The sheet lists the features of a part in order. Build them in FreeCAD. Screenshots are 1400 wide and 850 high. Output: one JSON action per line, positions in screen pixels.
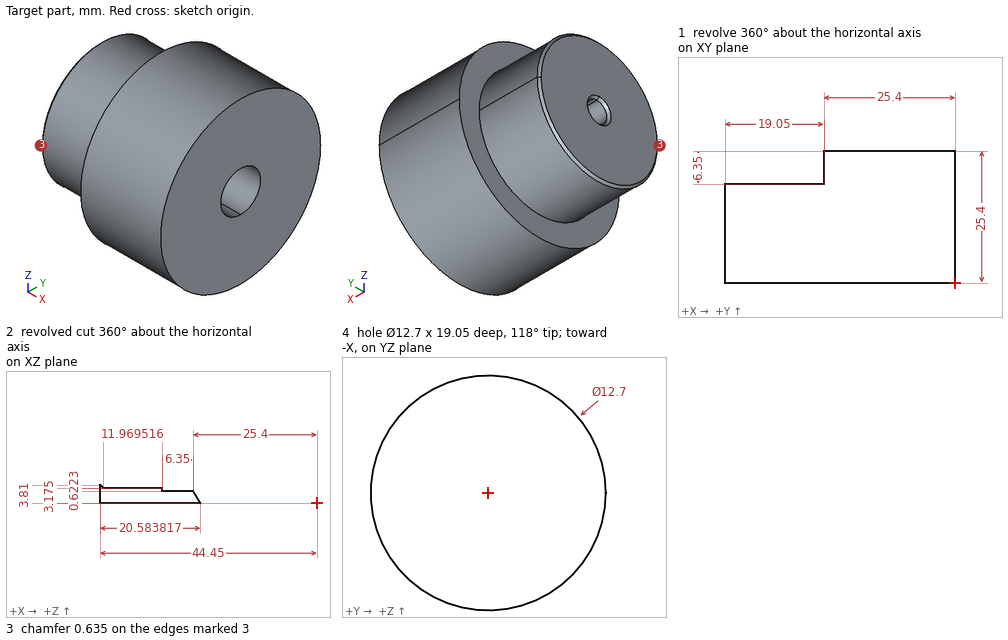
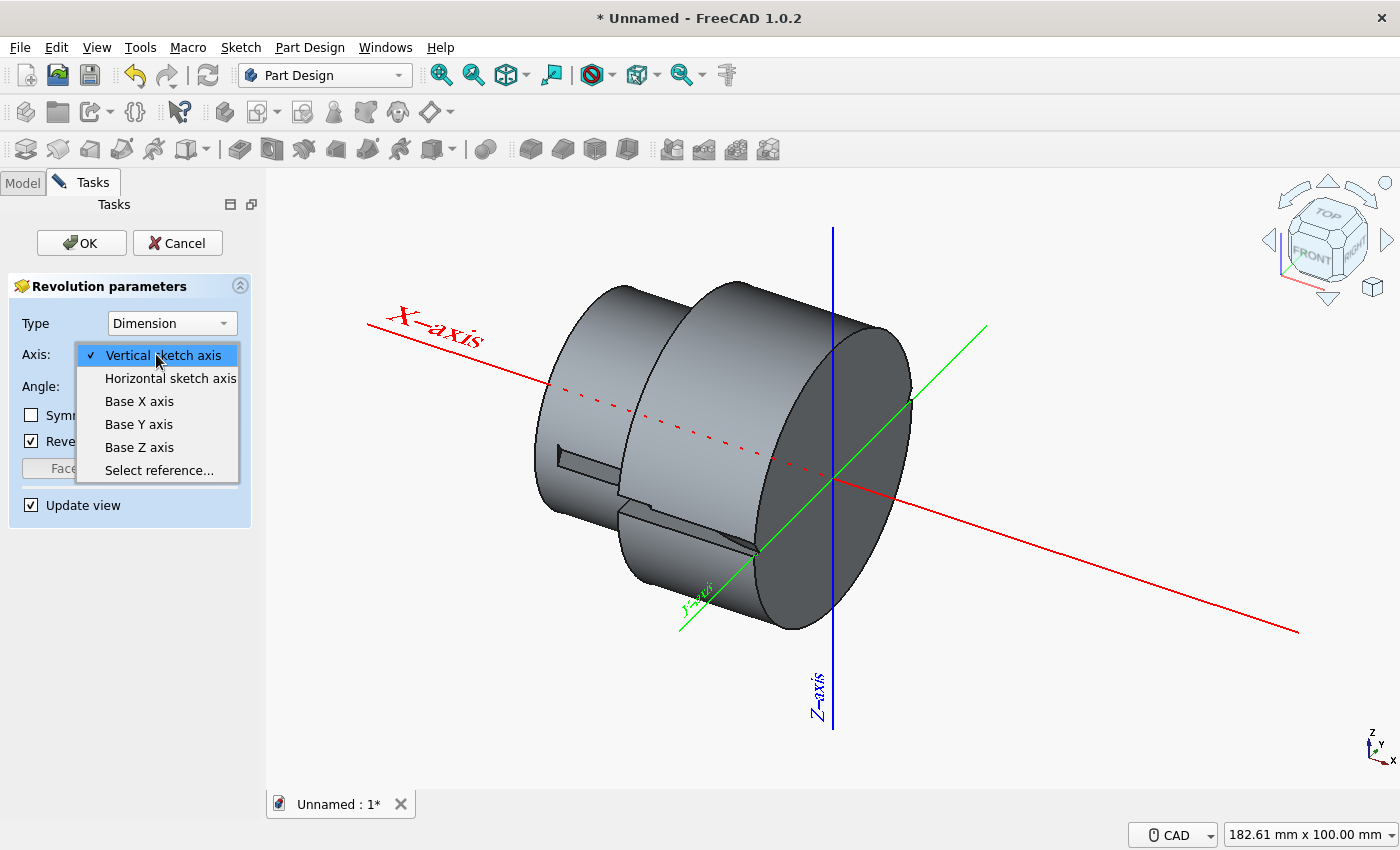
{"action": "left_click", "coordinate": [156, 378]}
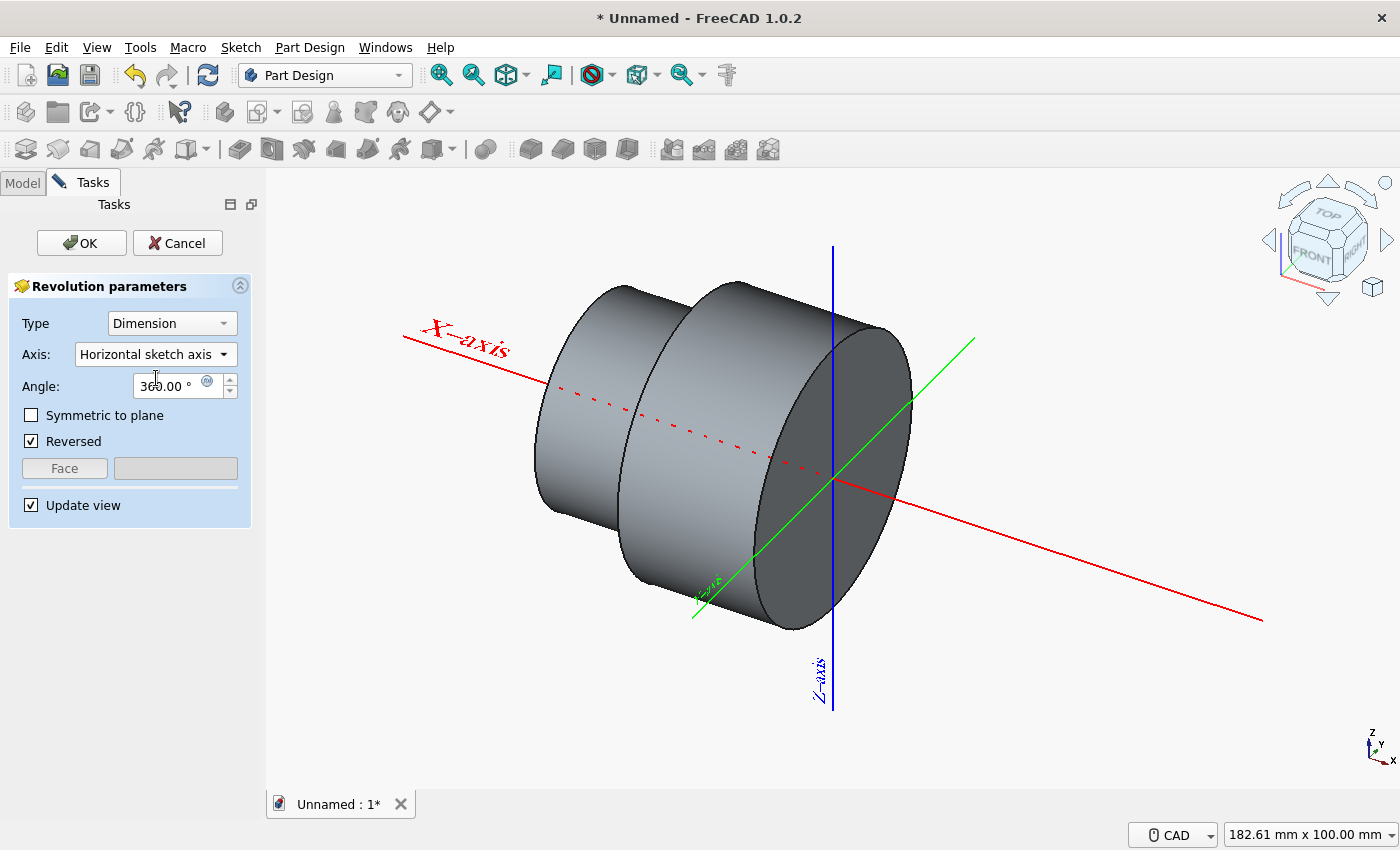
{"action": "left_click", "coordinate": [82, 243]}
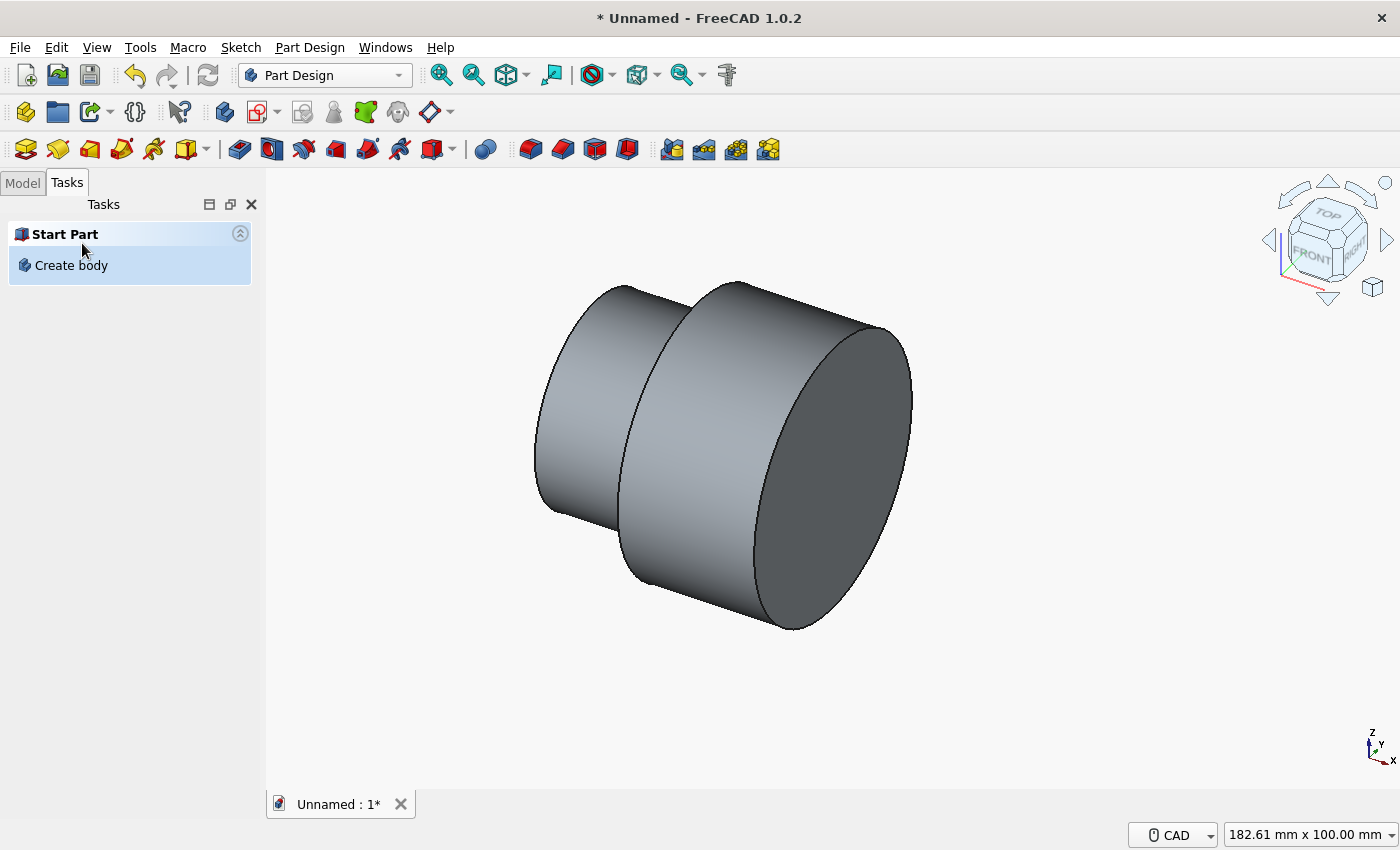
{"action": "key", "text": "0"}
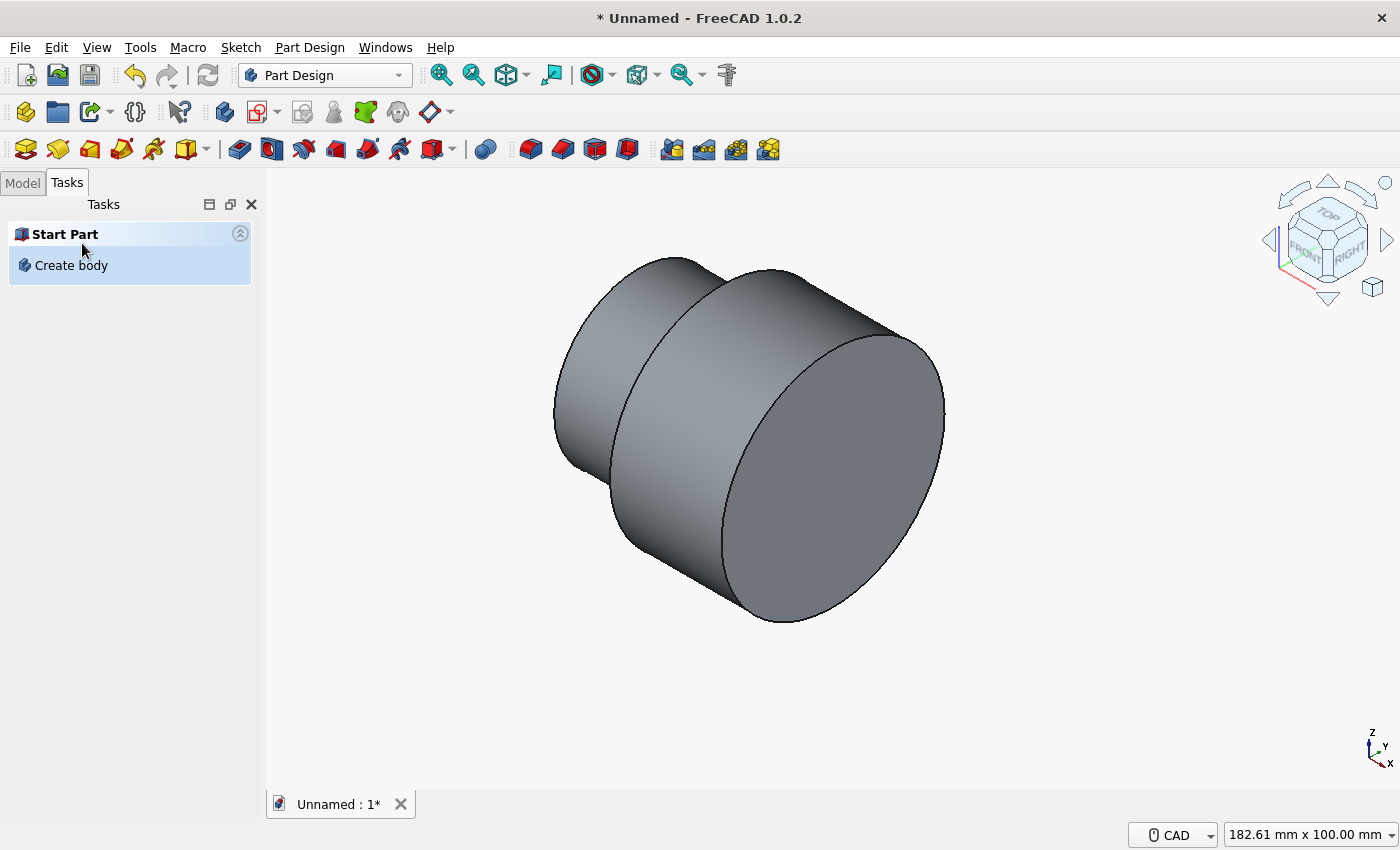
{"action": "key", "text": "2"}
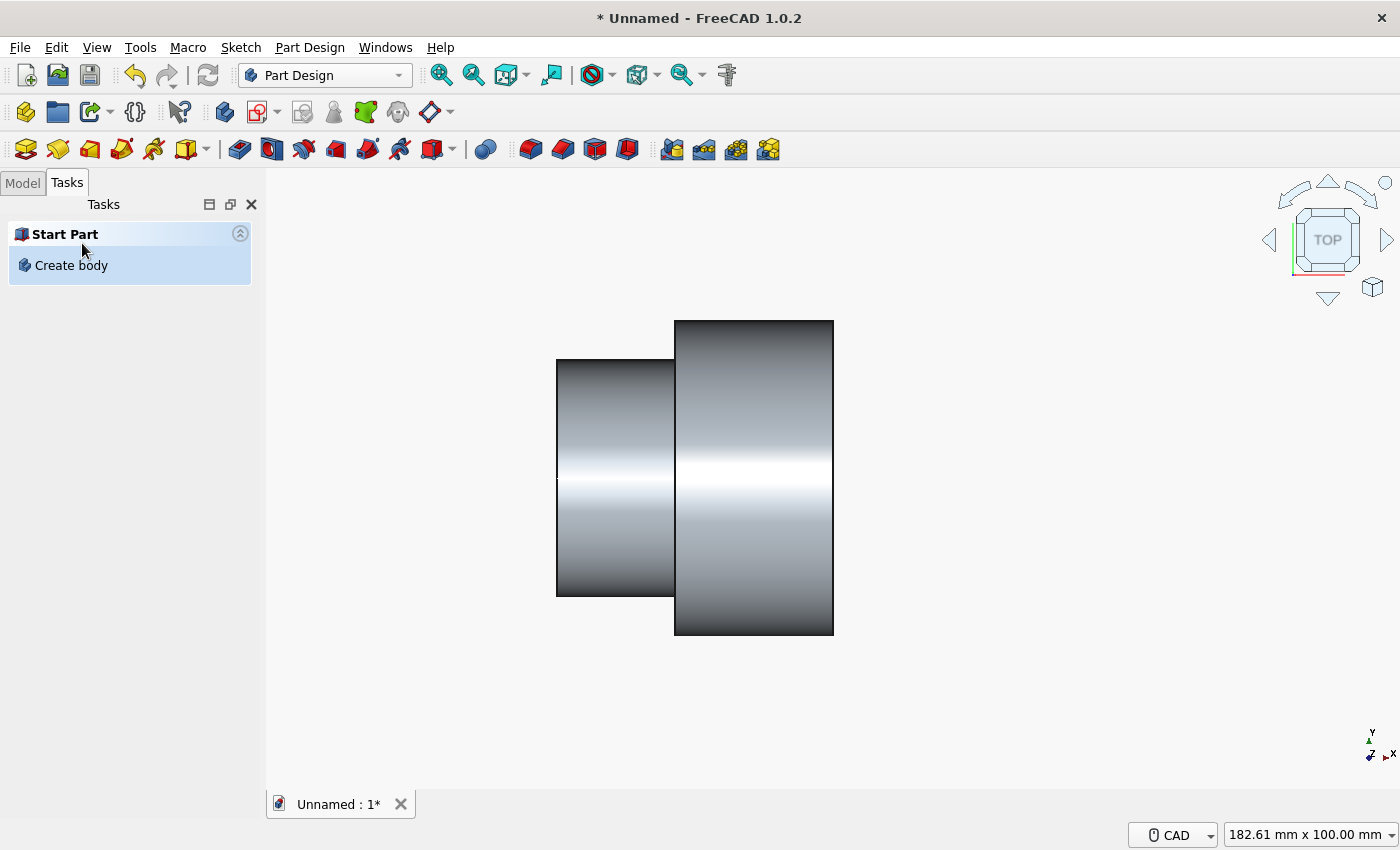
{"action": "left_click", "coordinate": [557, 573]}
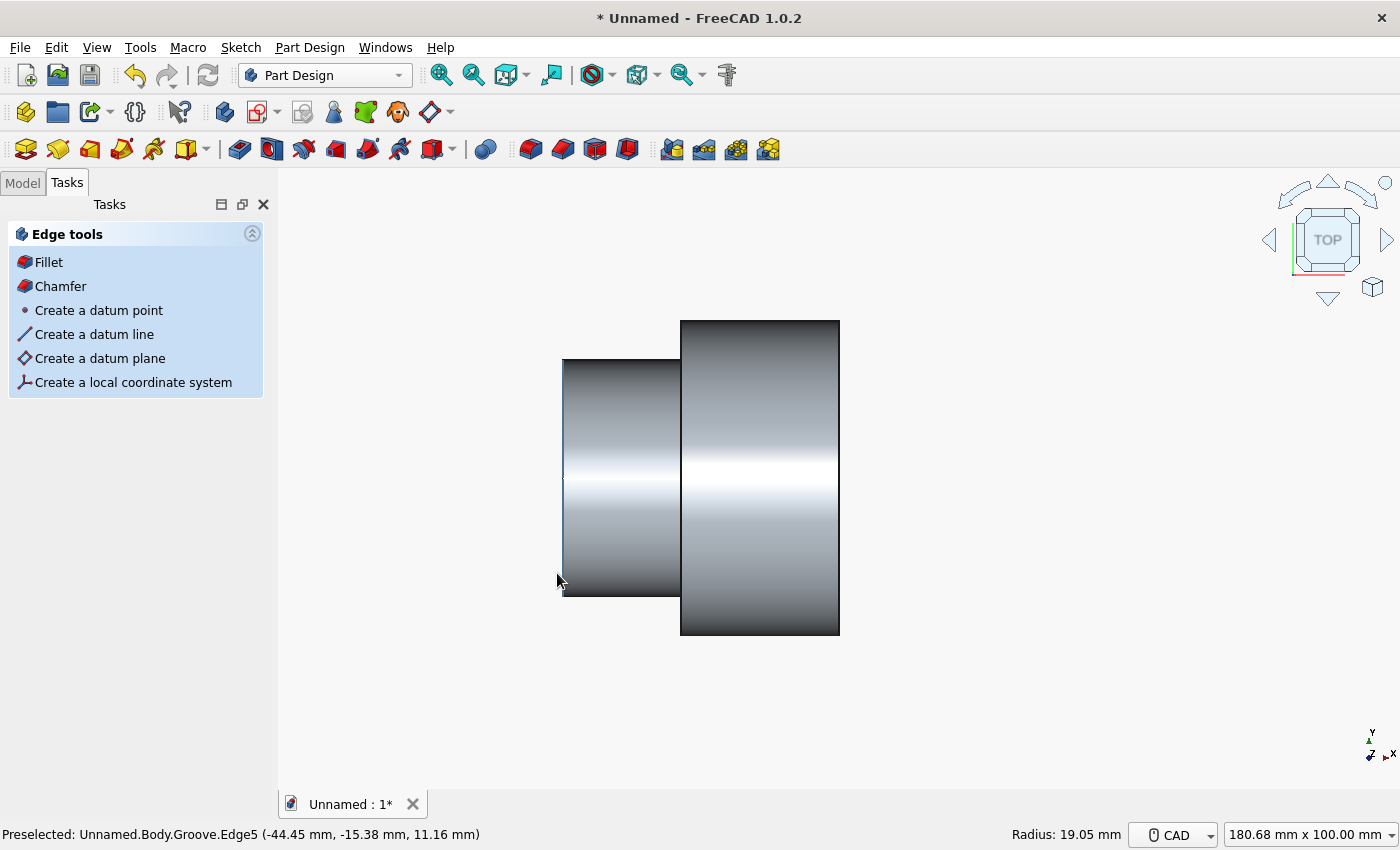
{"action": "left_click", "coordinate": [564, 150]}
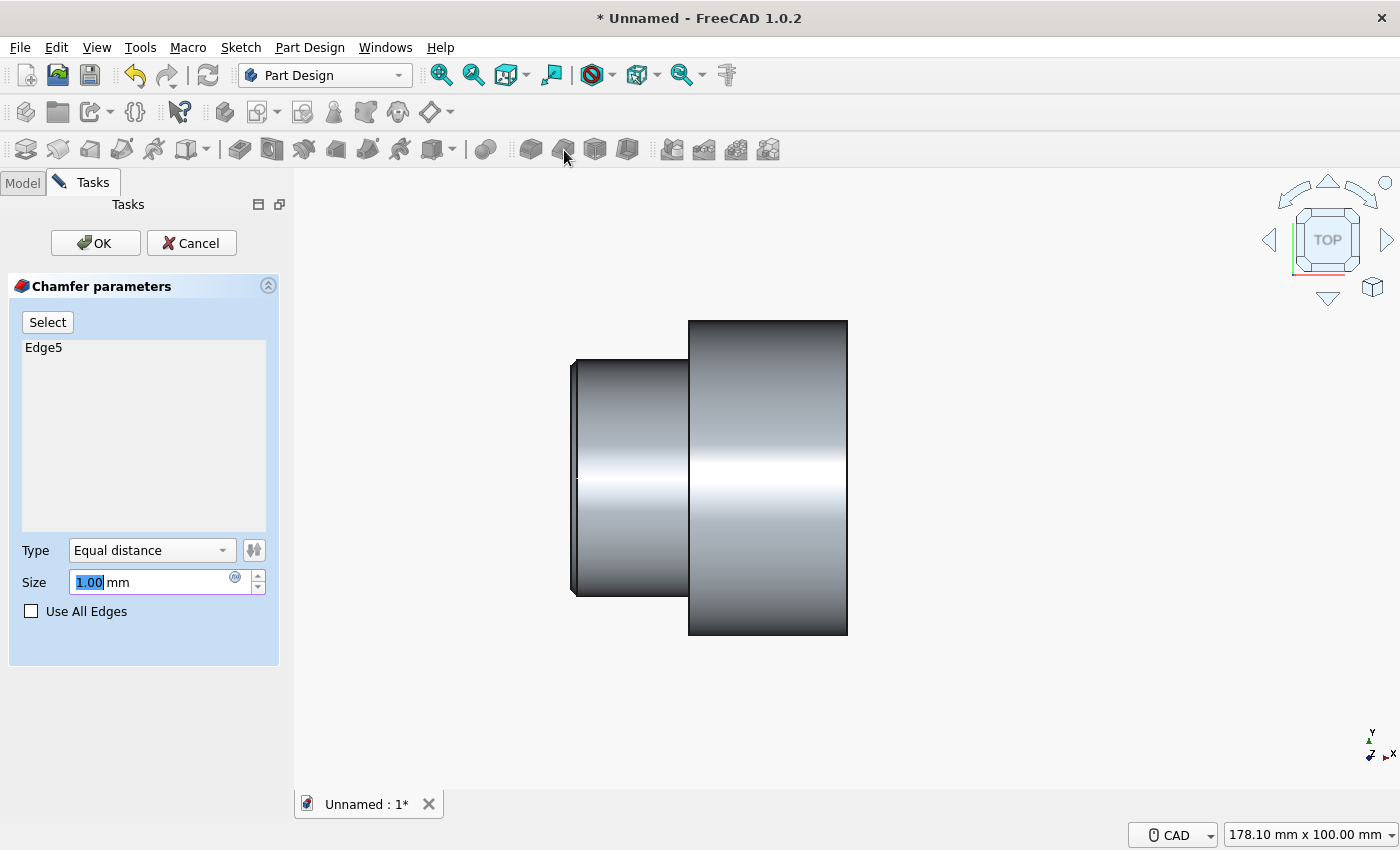
{"action": "type", "text": "0.635"}
{"action": "key", "text": "Tab"}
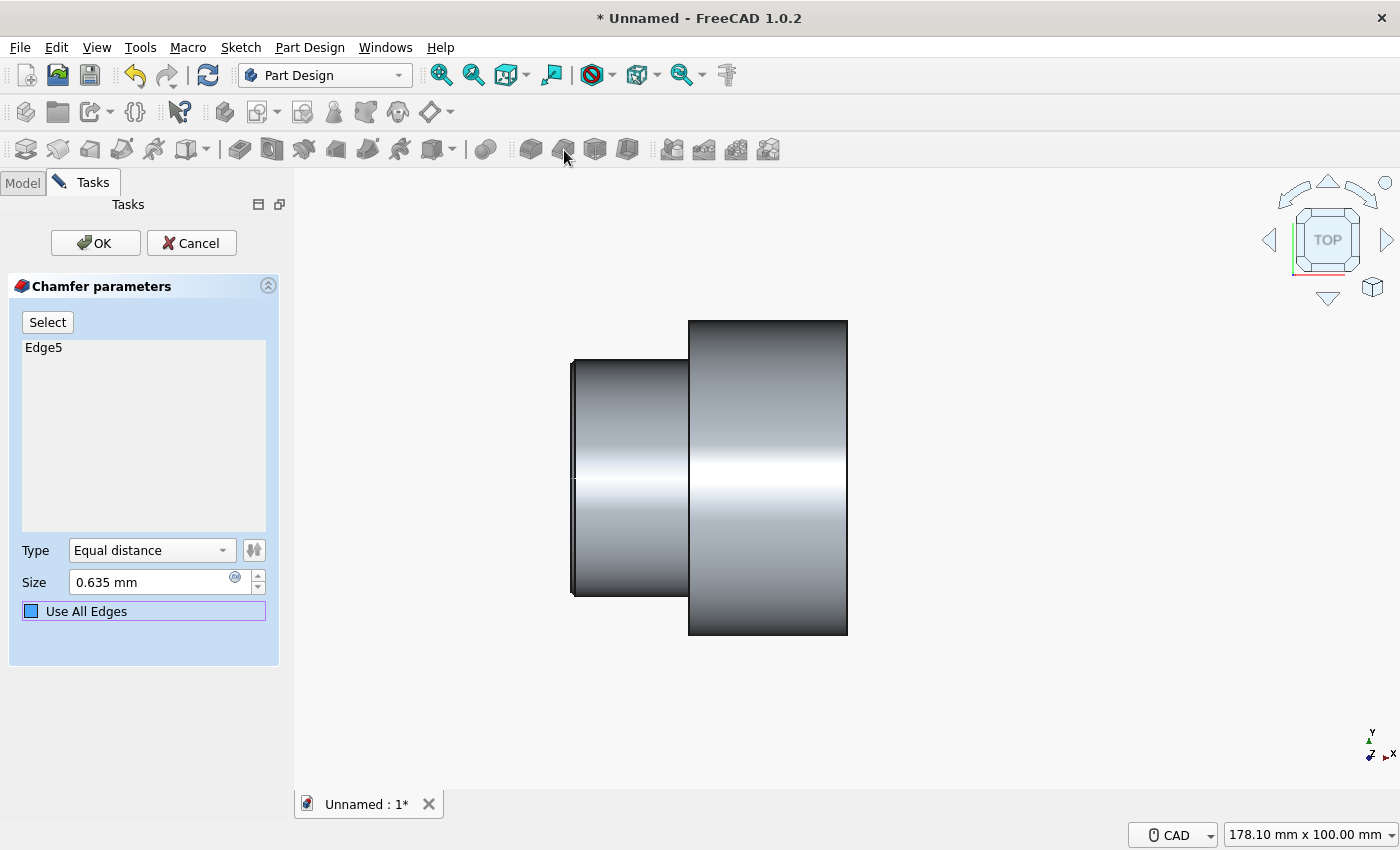
{"action": "left_click", "coordinate": [96, 243]}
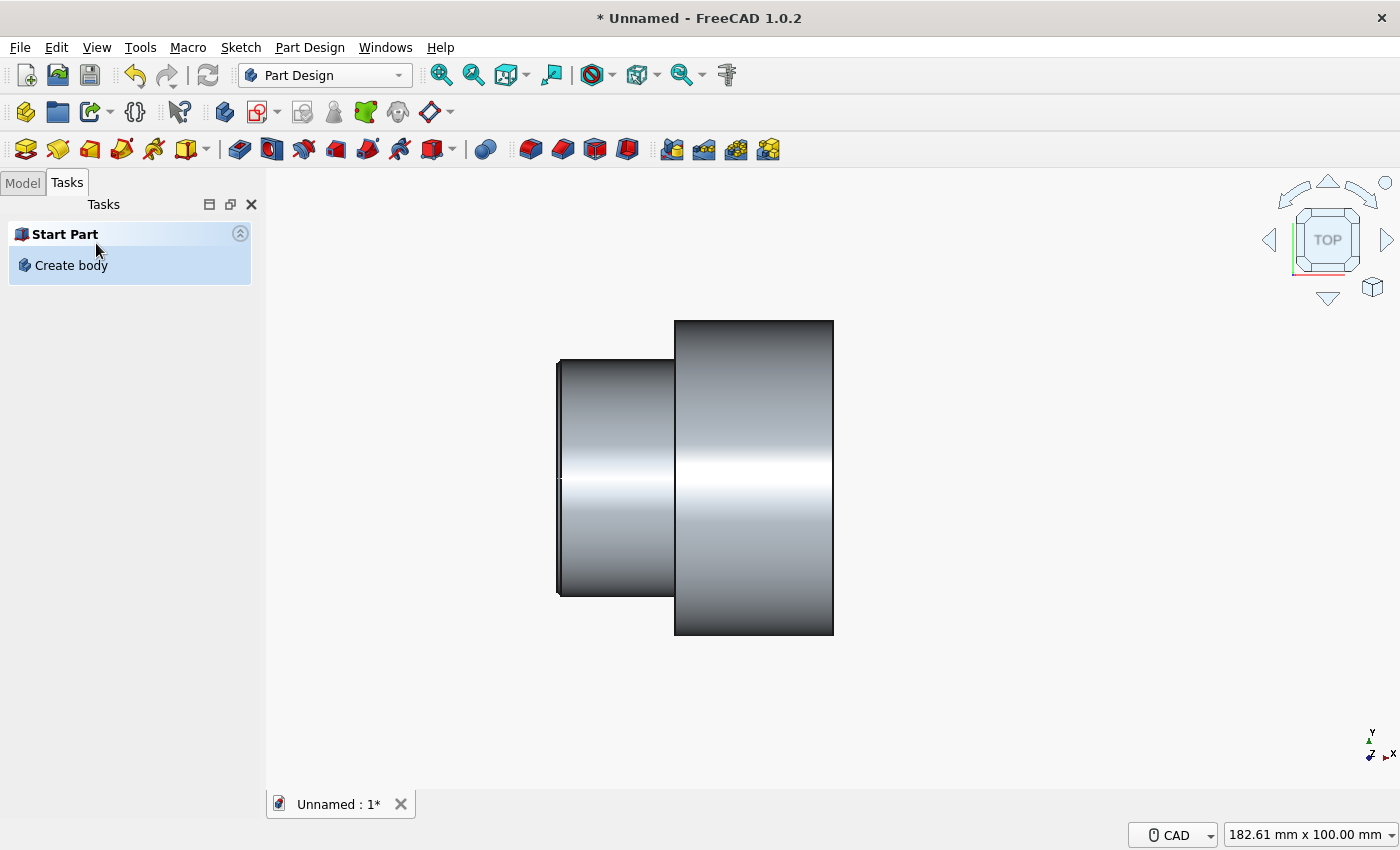
{"action": "left_click", "coordinate": [258, 112]}